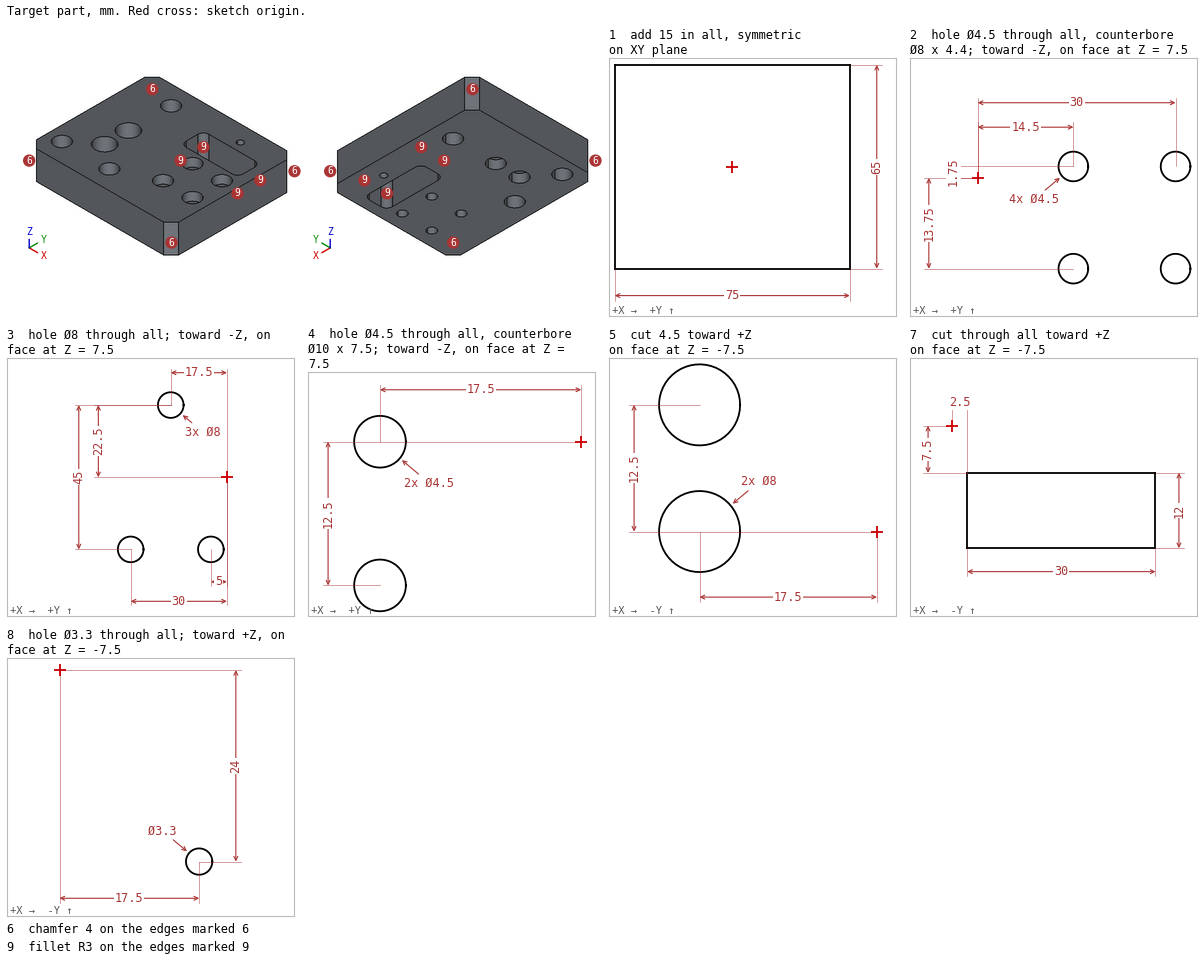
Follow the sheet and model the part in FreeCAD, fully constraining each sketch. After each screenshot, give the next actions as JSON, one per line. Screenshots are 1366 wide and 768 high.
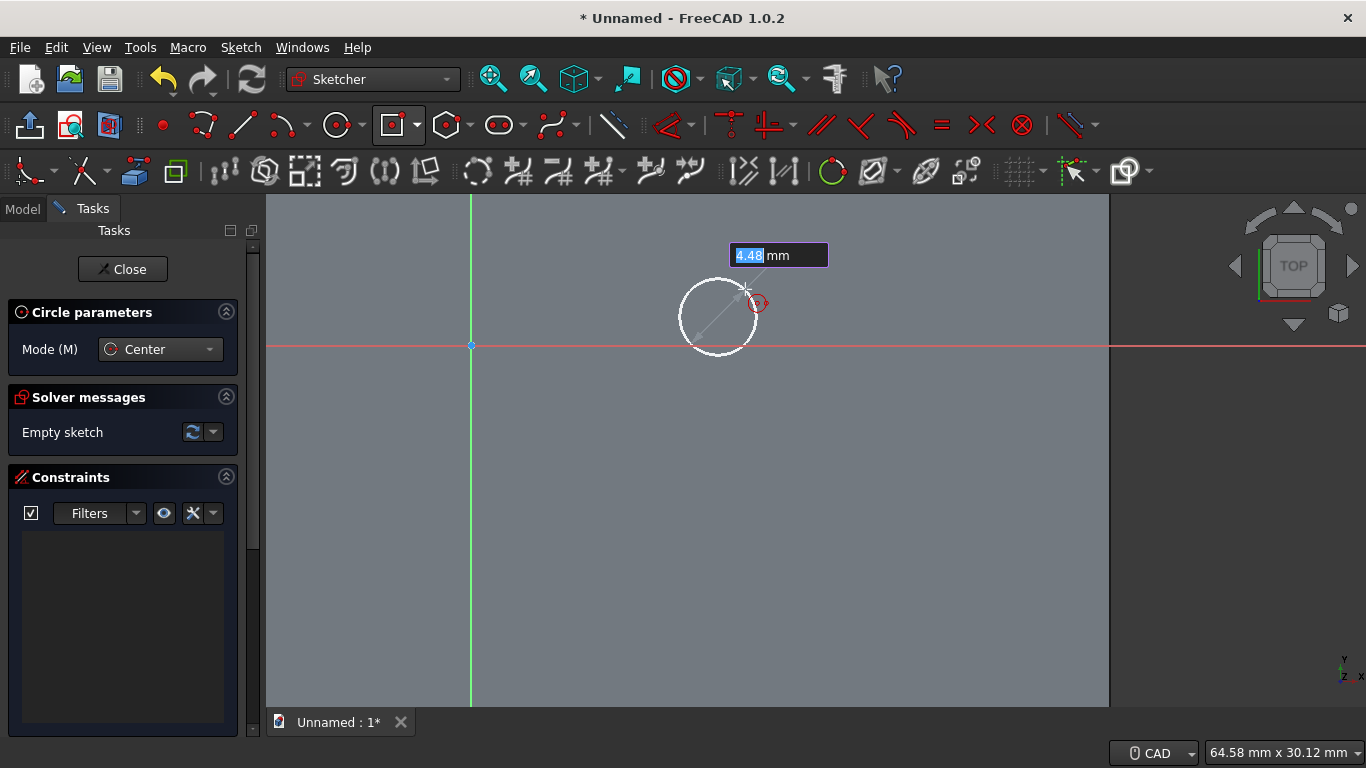
{"action": "type", "text": "4.5"}
{"action": "key", "text": "Return"}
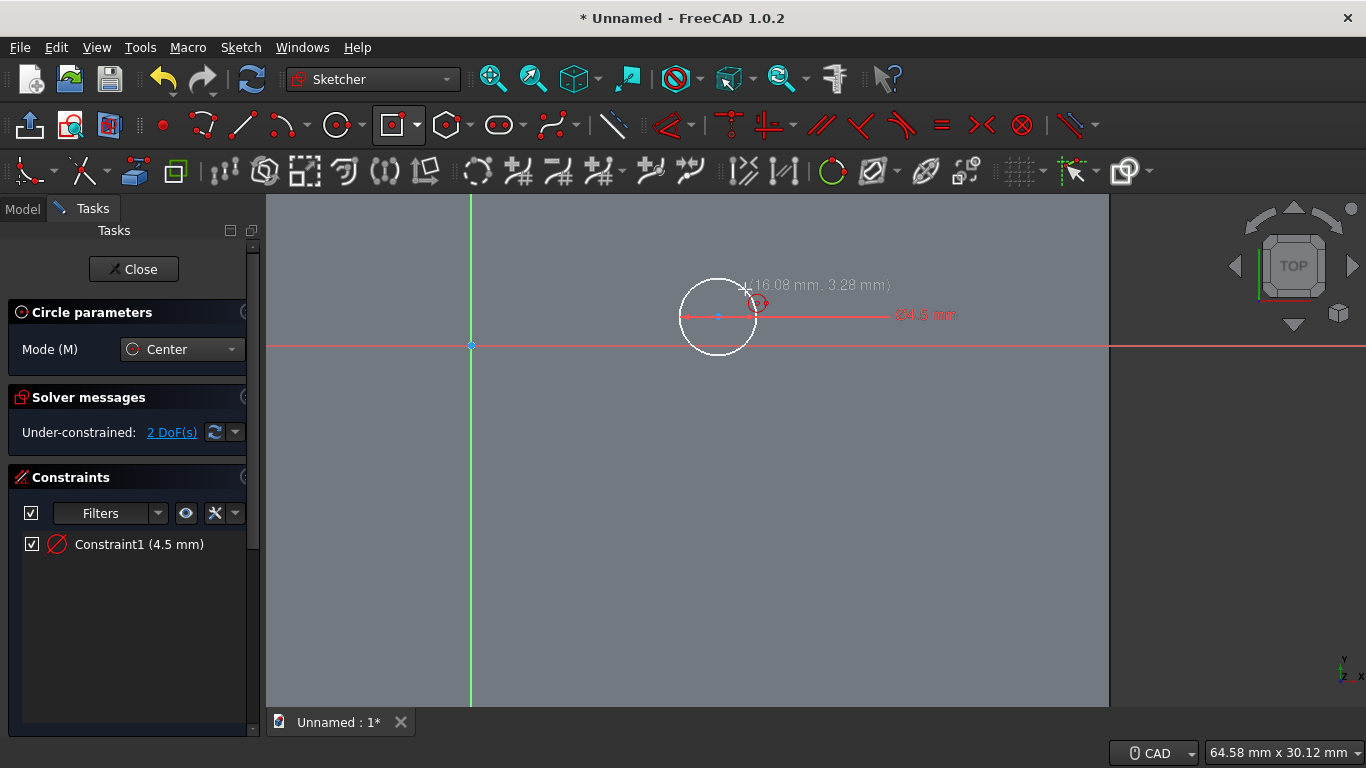
{"action": "left_click", "coordinate": [718, 580]}
{"action": "mouse_move", "coordinate": [745, 553]}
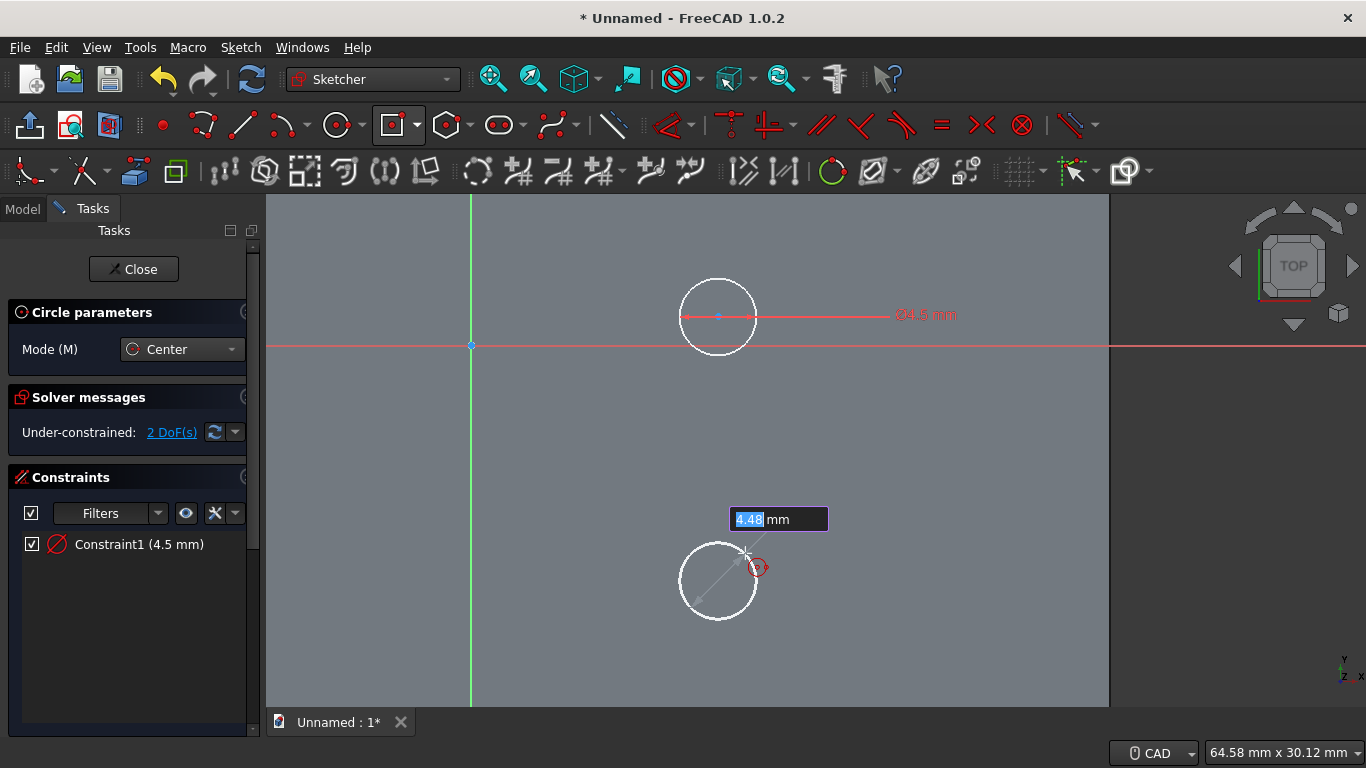
{"action": "type", "text": "4.5"}
{"action": "key", "text": "Return"}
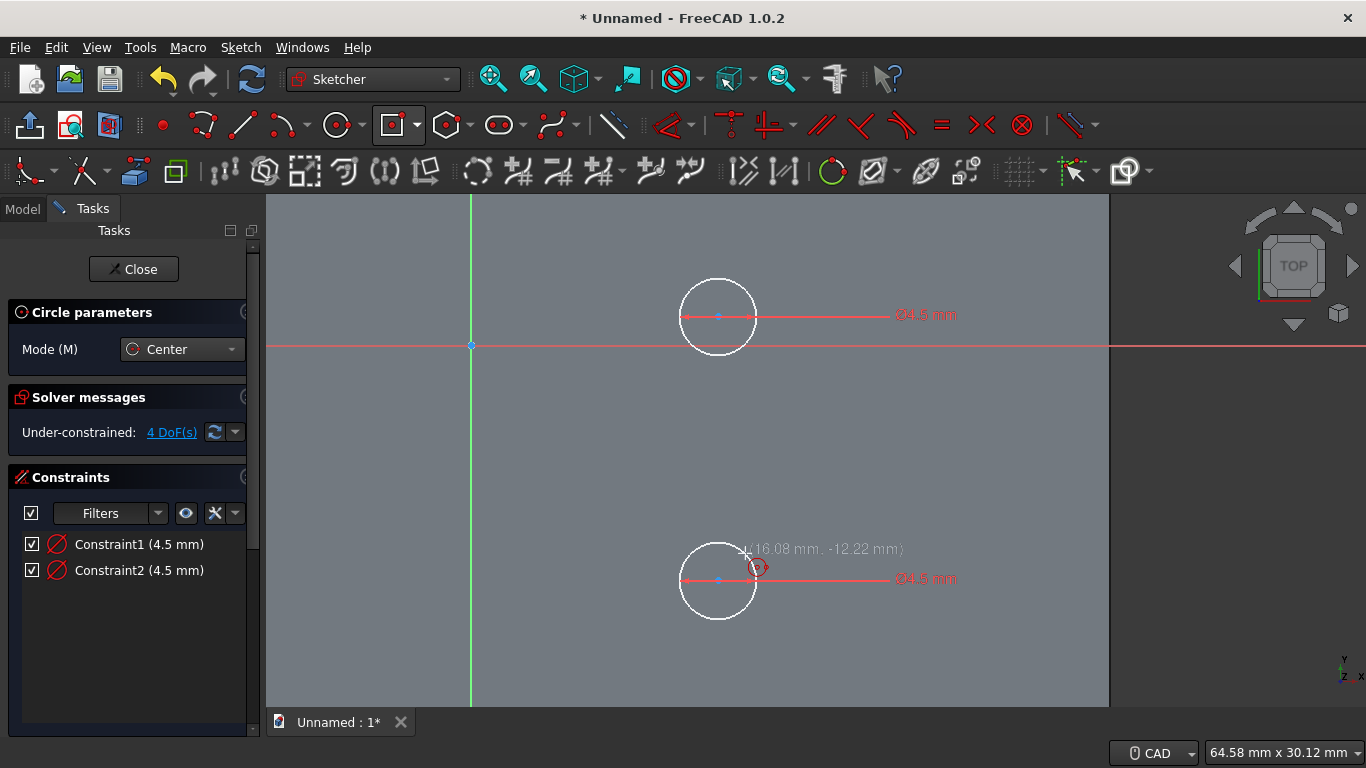
{"action": "left_click", "coordinate": [982, 316]}
{"action": "mouse_move", "coordinate": [1009, 289]}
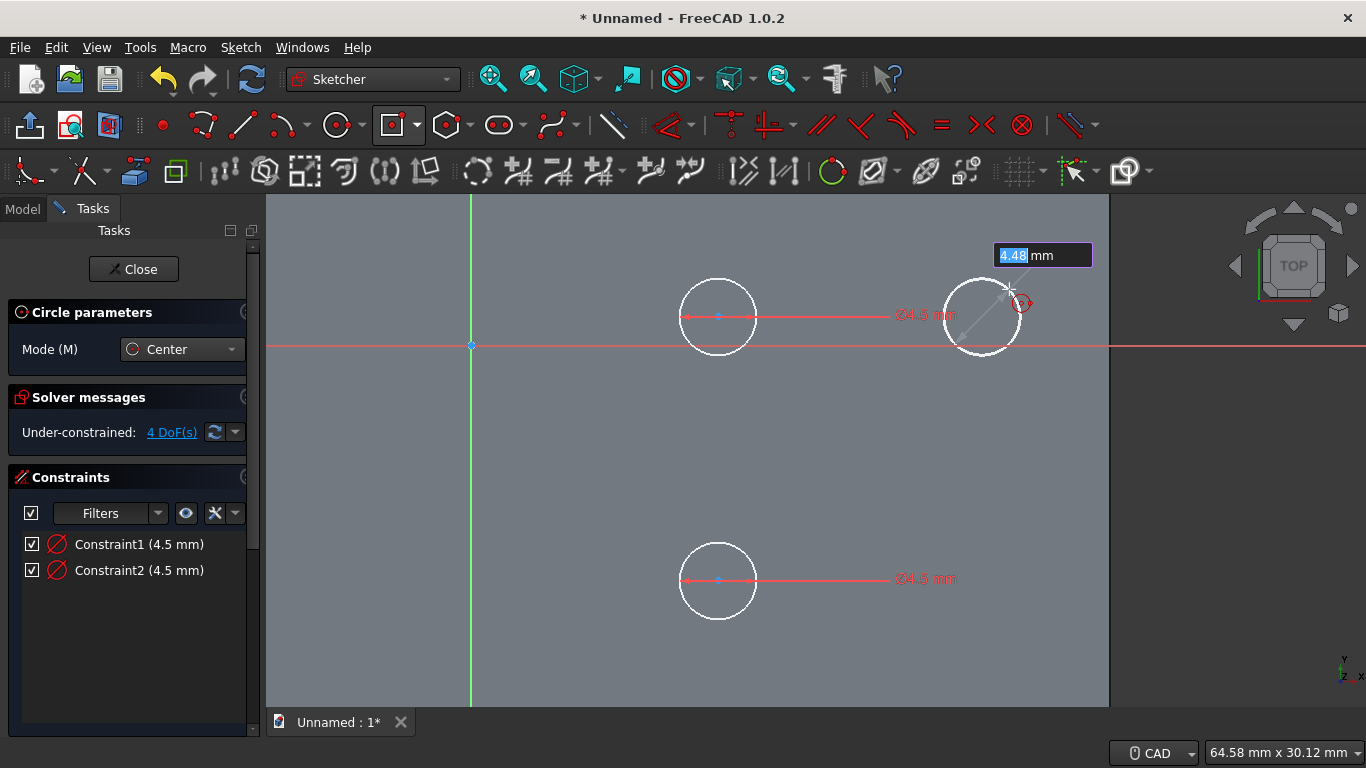
{"action": "type", "text": "4.5"}
{"action": "key", "text": "Return"}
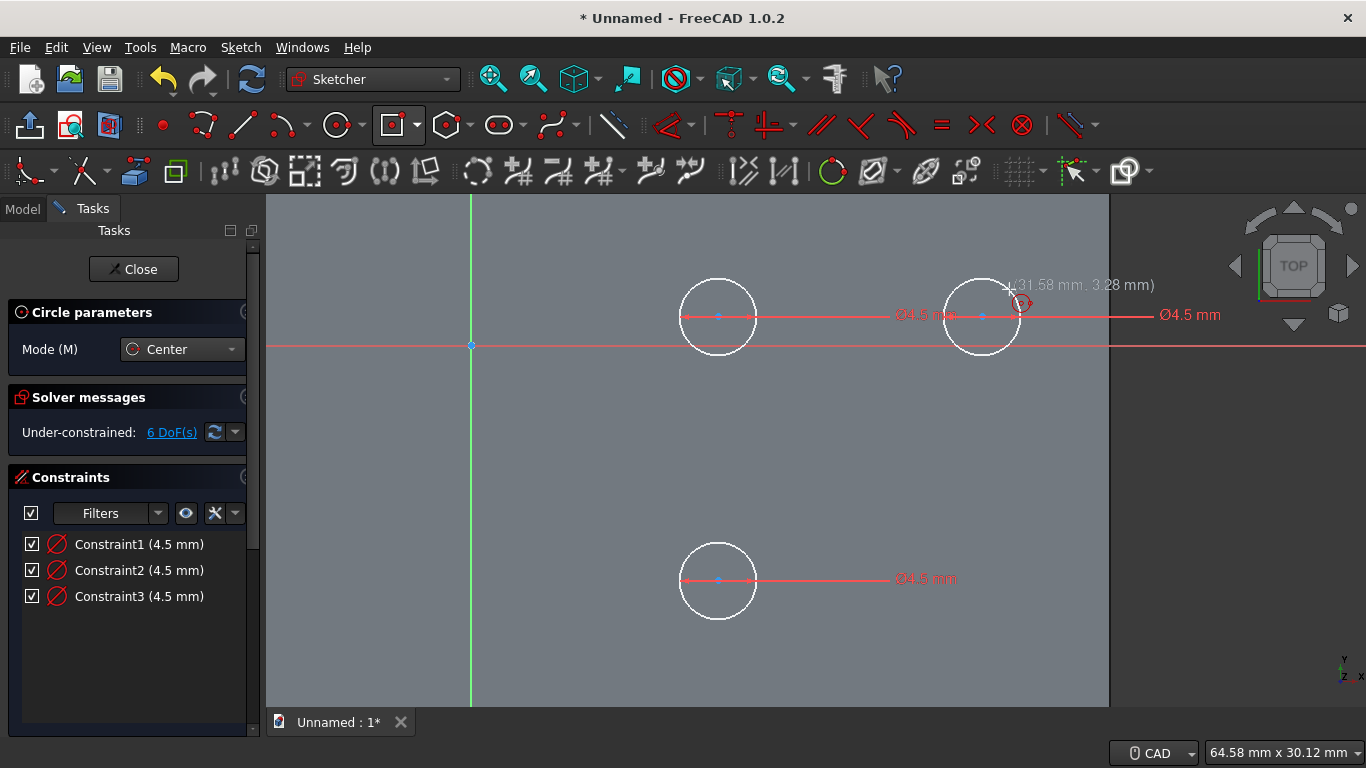
{"action": "left_click", "coordinate": [982, 580]}
{"action": "mouse_move", "coordinate": [1009, 553]}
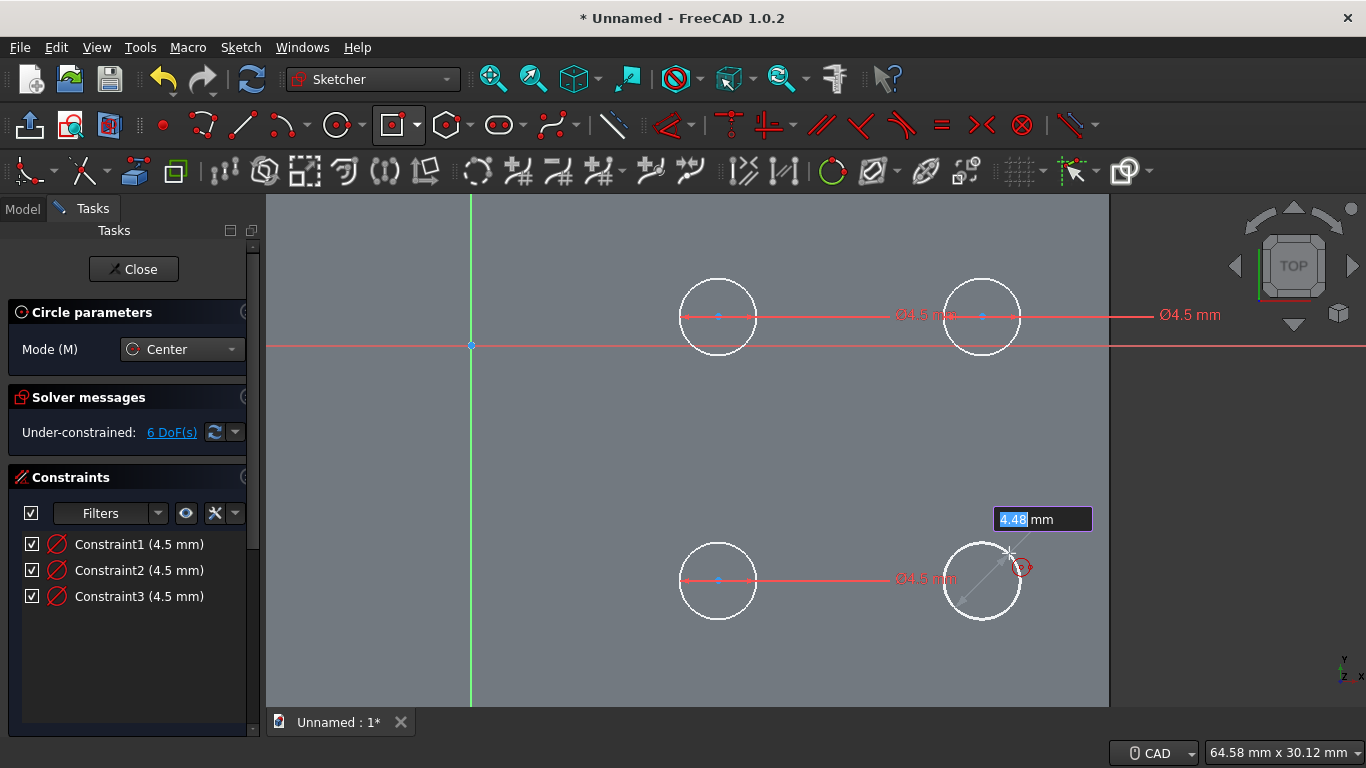
{"action": "type", "text": "4.5"}
{"action": "key", "text": "Return"}
{"action": "key", "text": "Escape"}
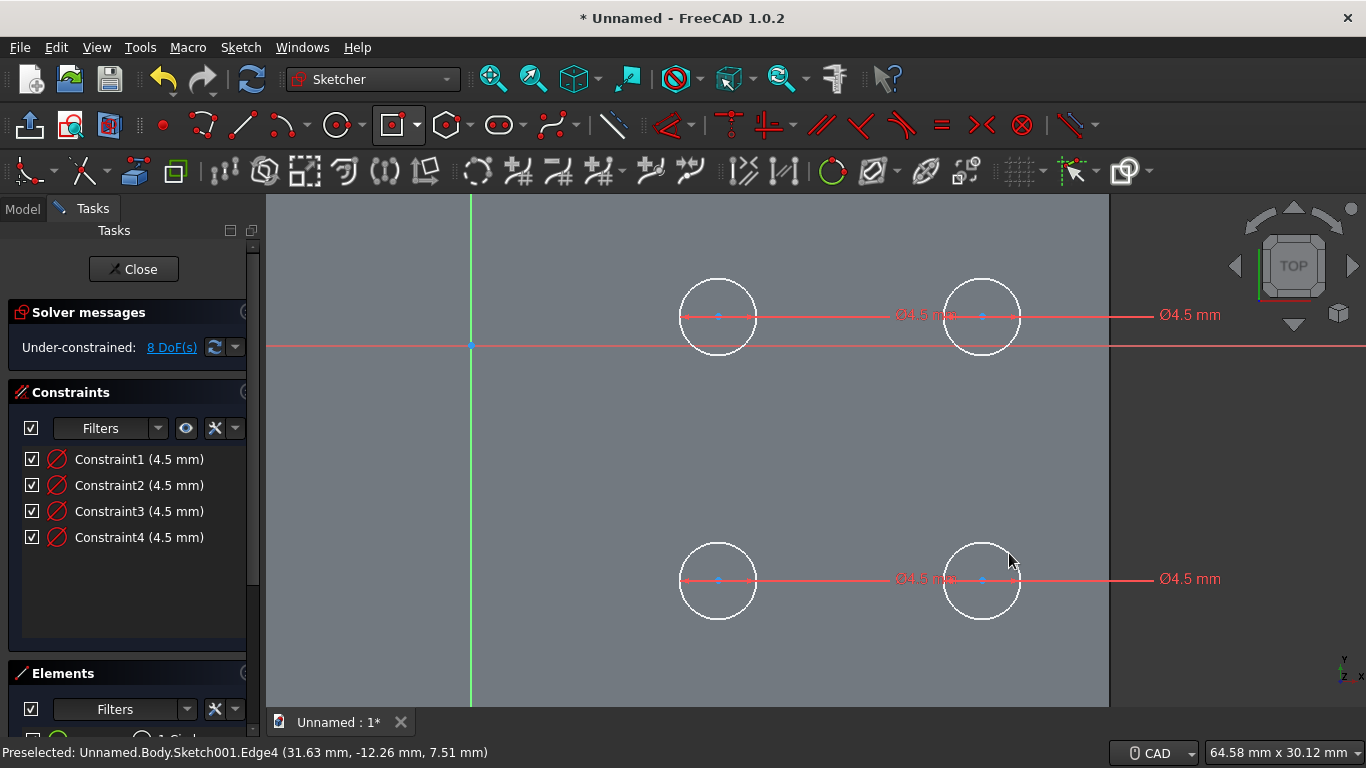
{"action": "left_click", "coordinate": [718, 317]}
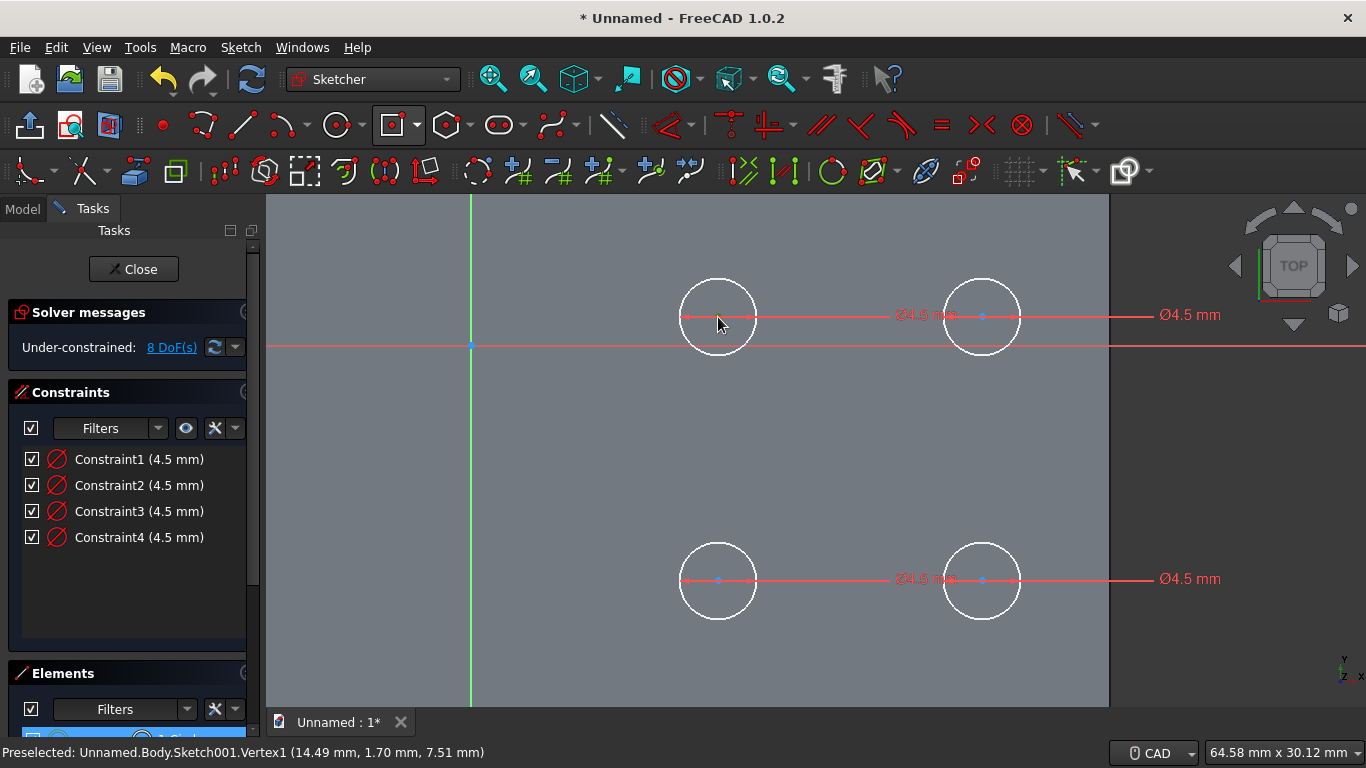
{"action": "left_click", "coordinate": [718, 581]}